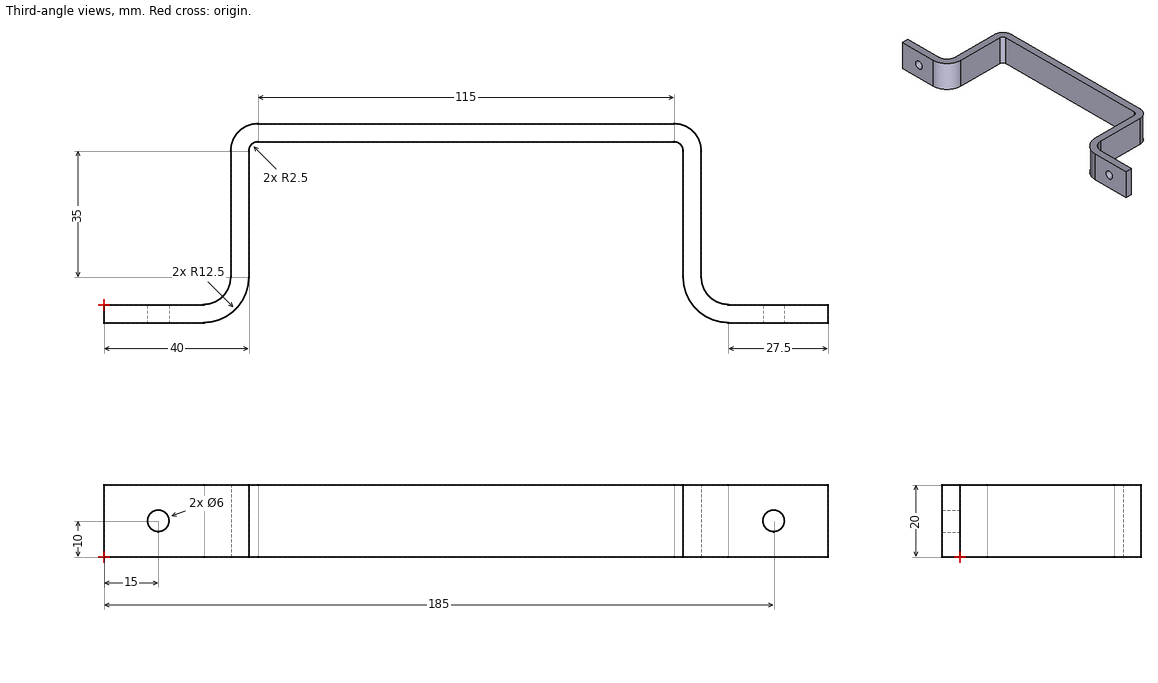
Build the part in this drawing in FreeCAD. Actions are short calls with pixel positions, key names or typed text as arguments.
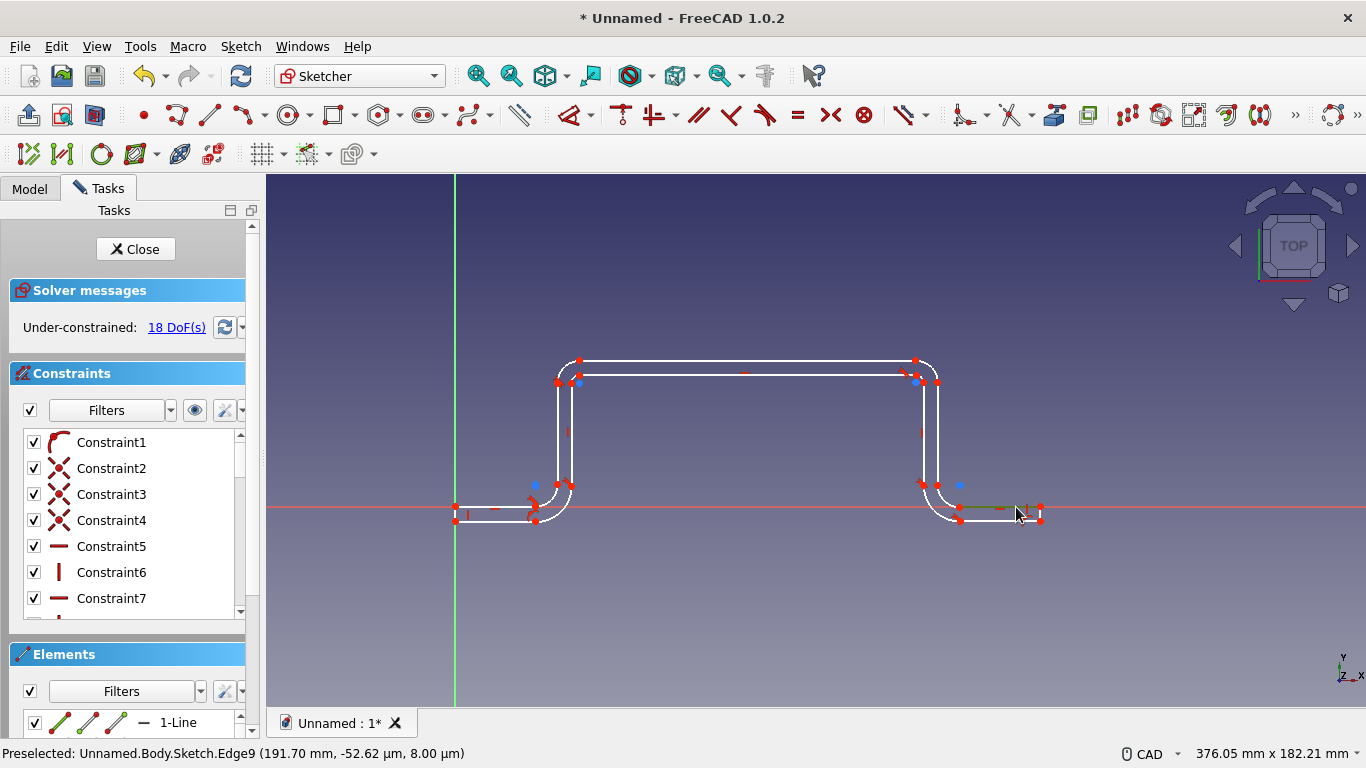
key(h)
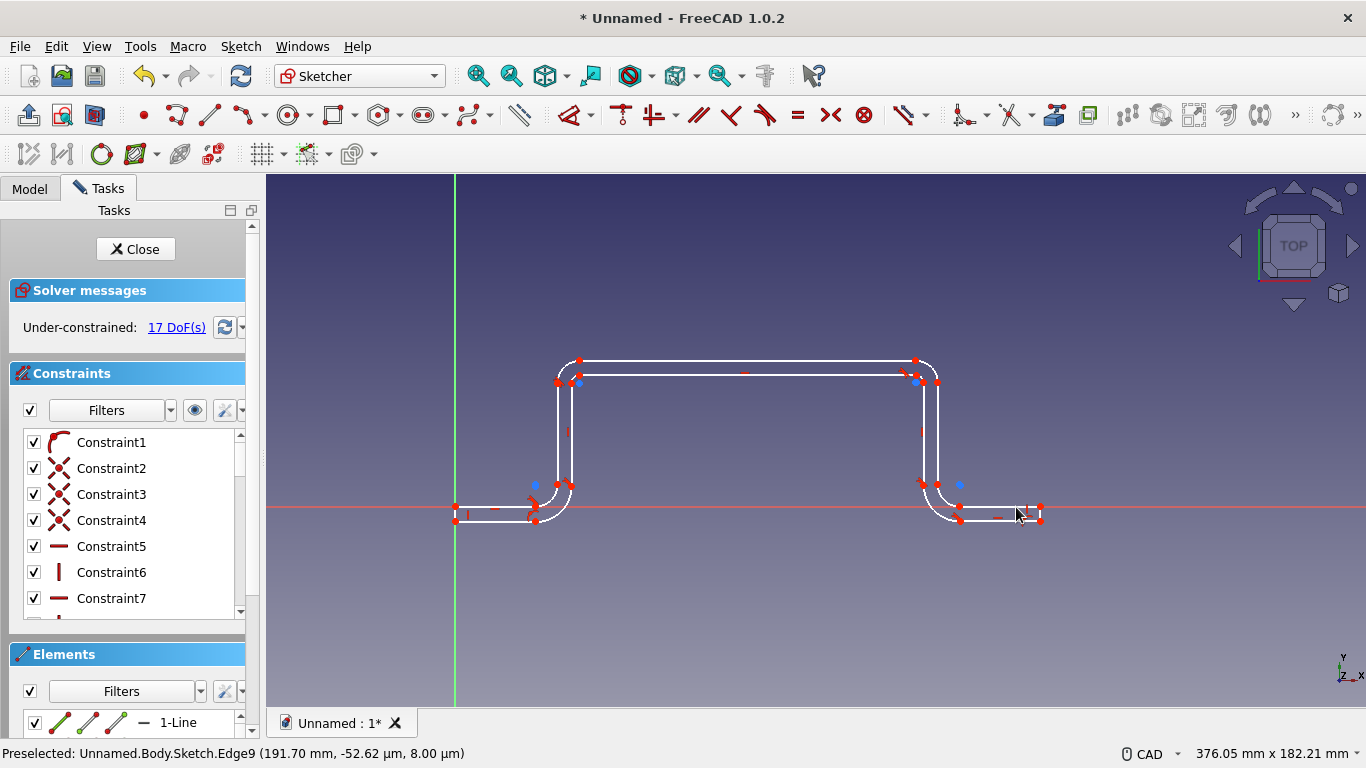
scroll(944, 518, up, 2)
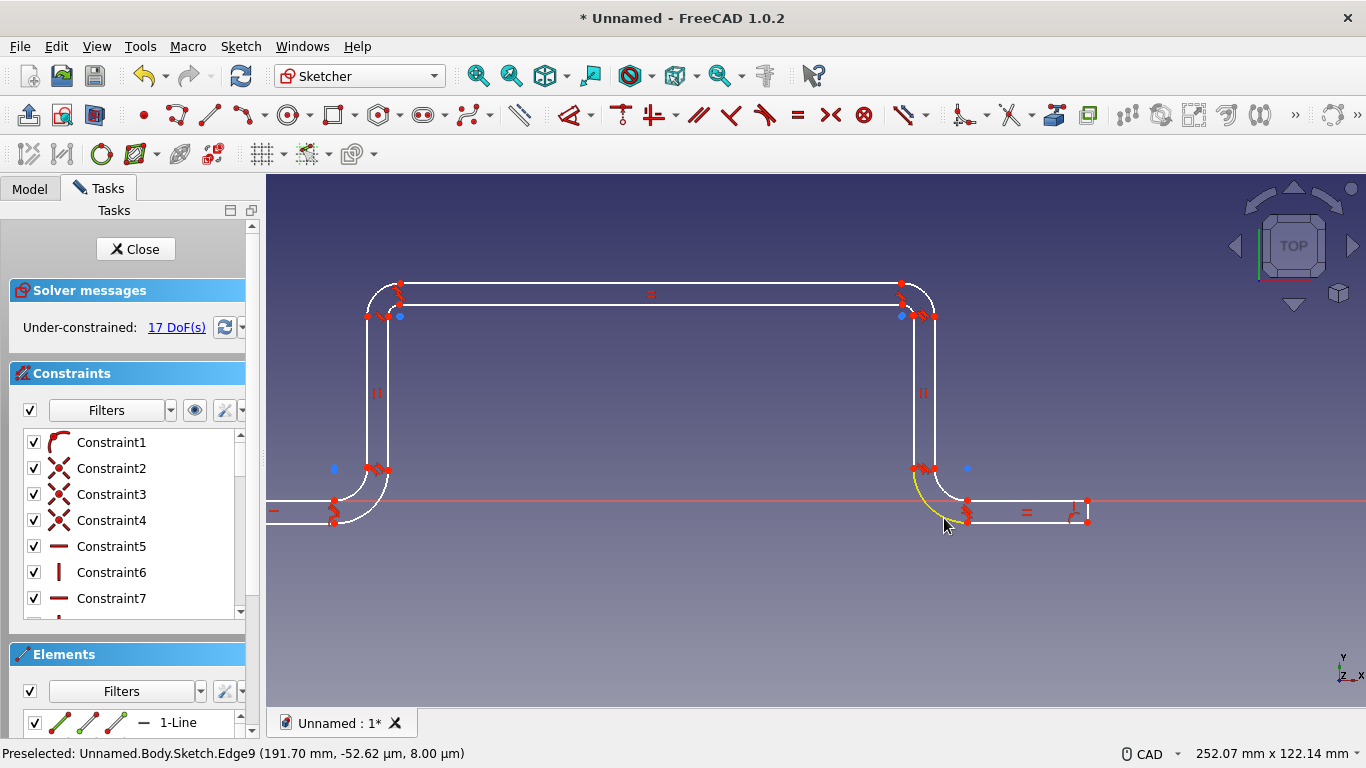
click(943, 517)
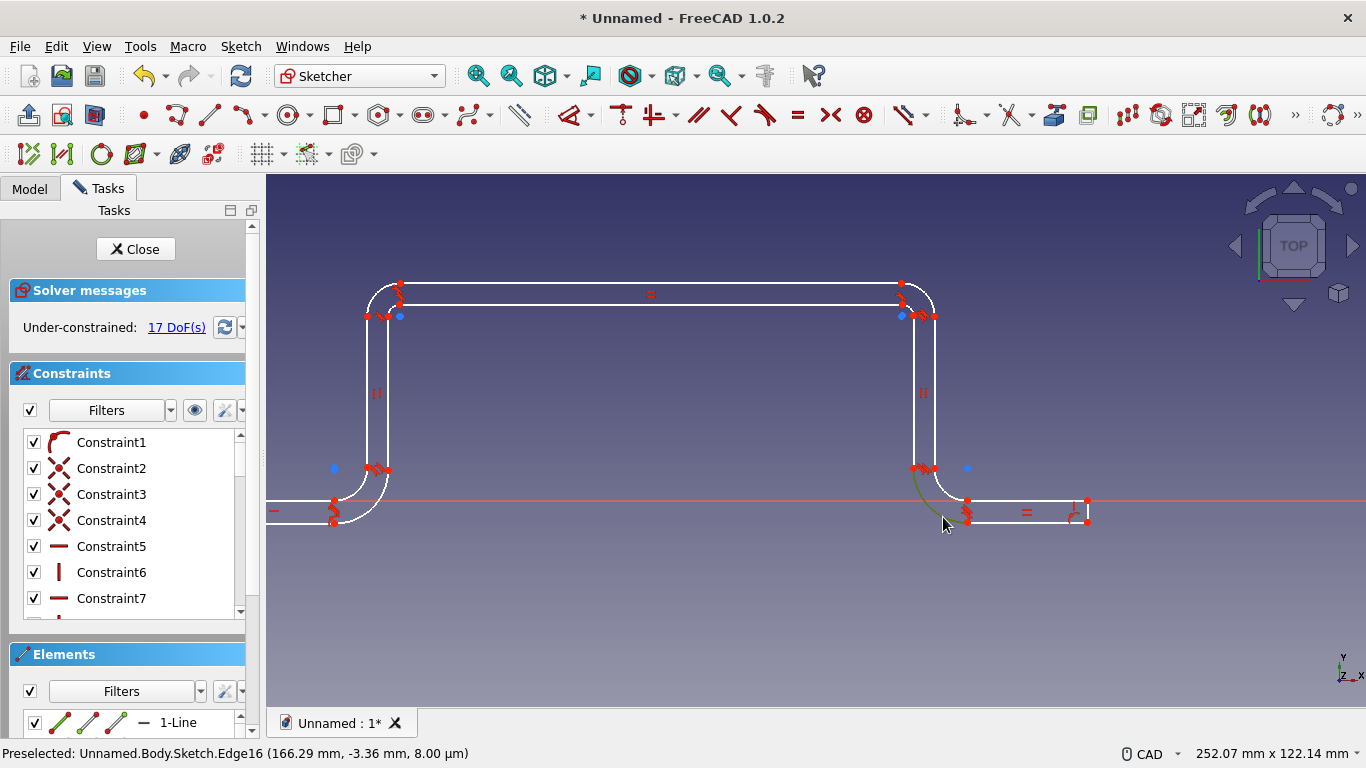
click(938, 483)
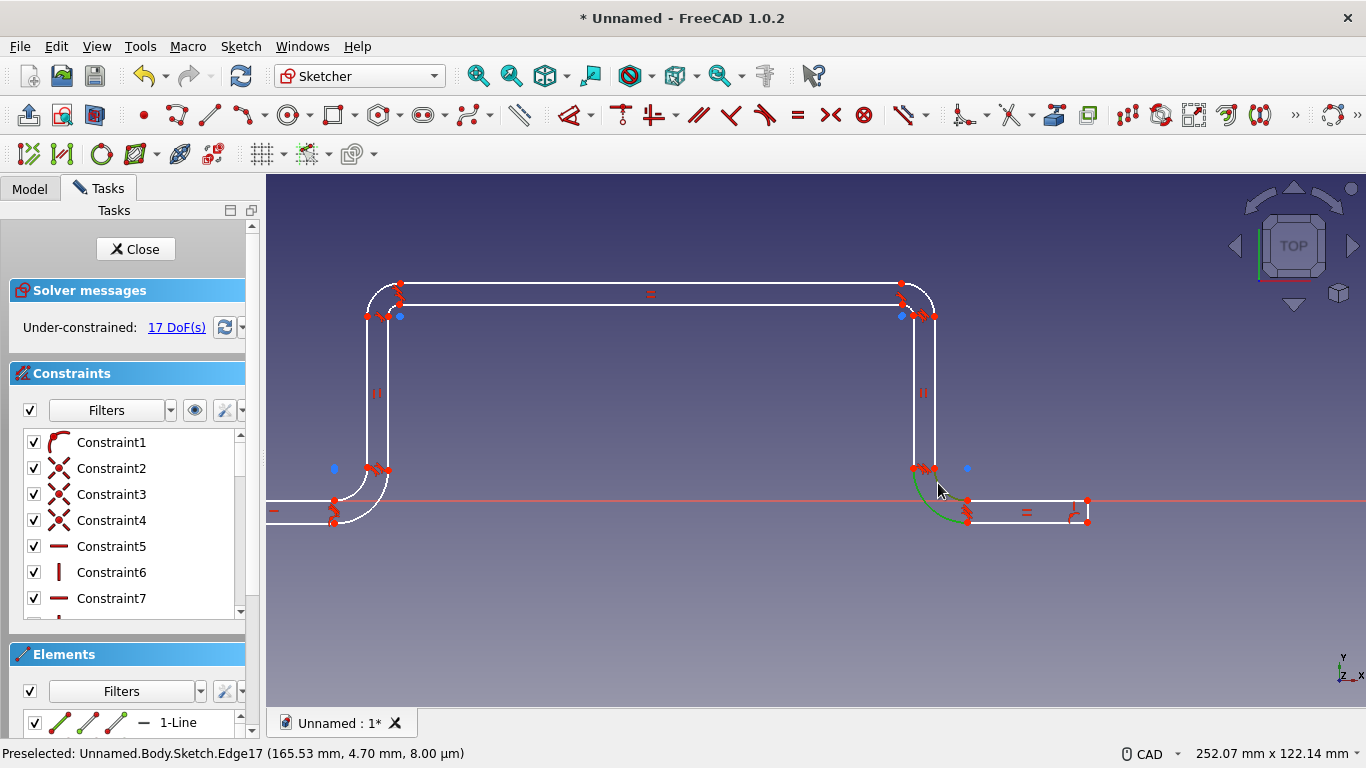
key(c)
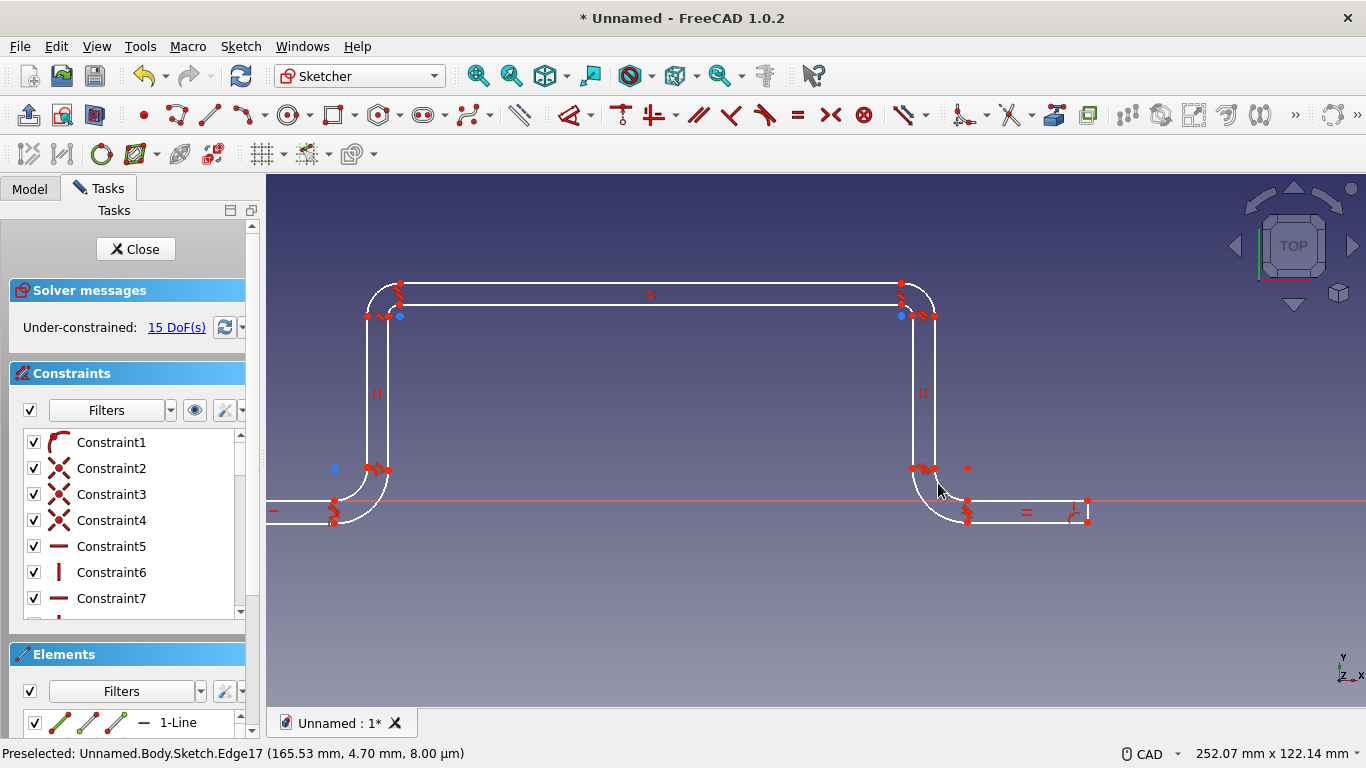
scroll(909, 308, up, 3)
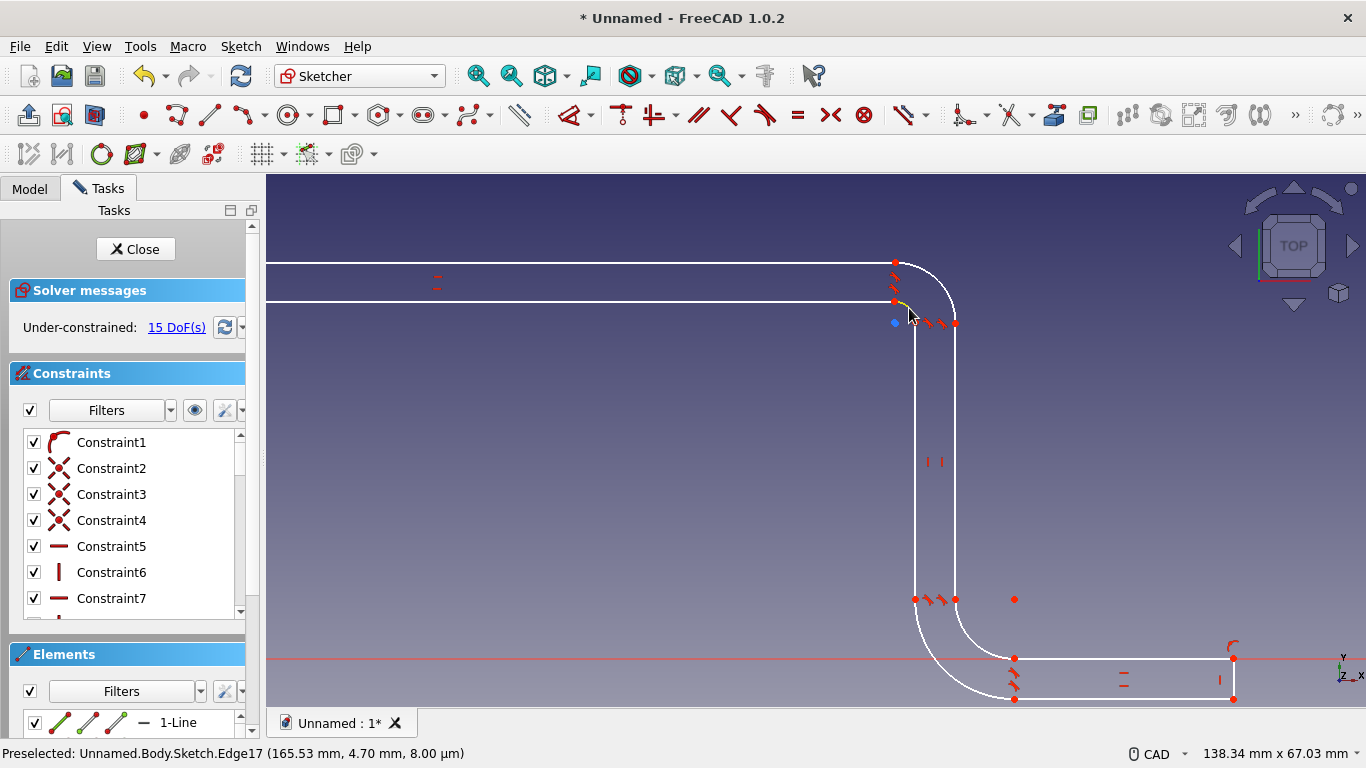
click(909, 308)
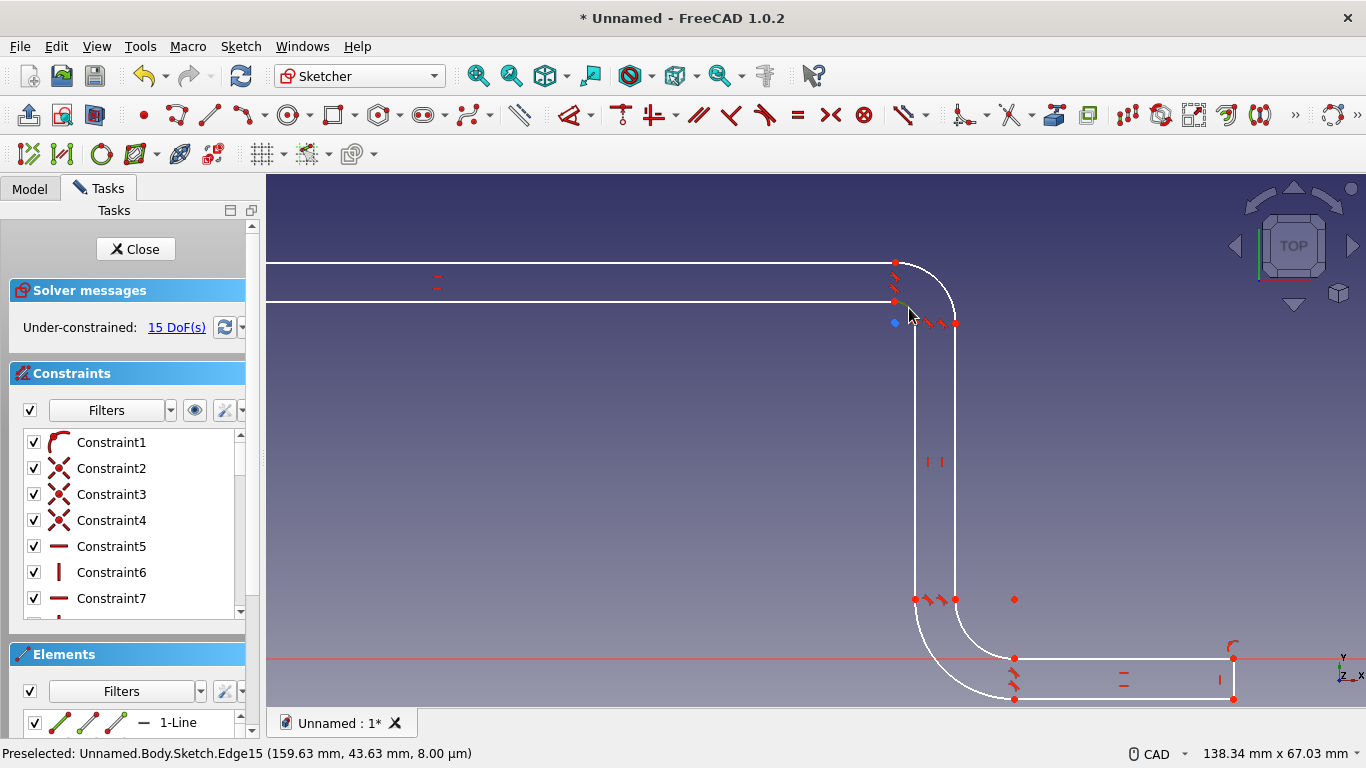
click(949, 296)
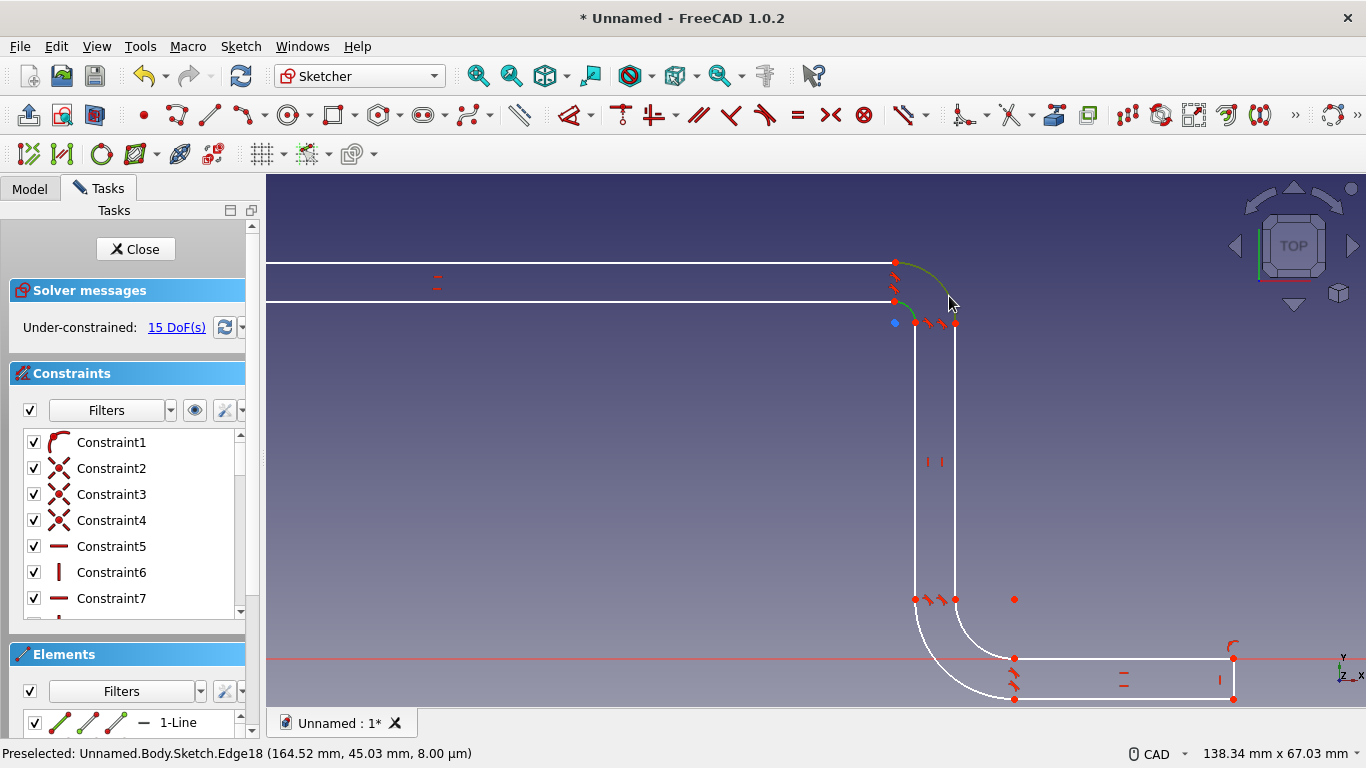
click(621, 116)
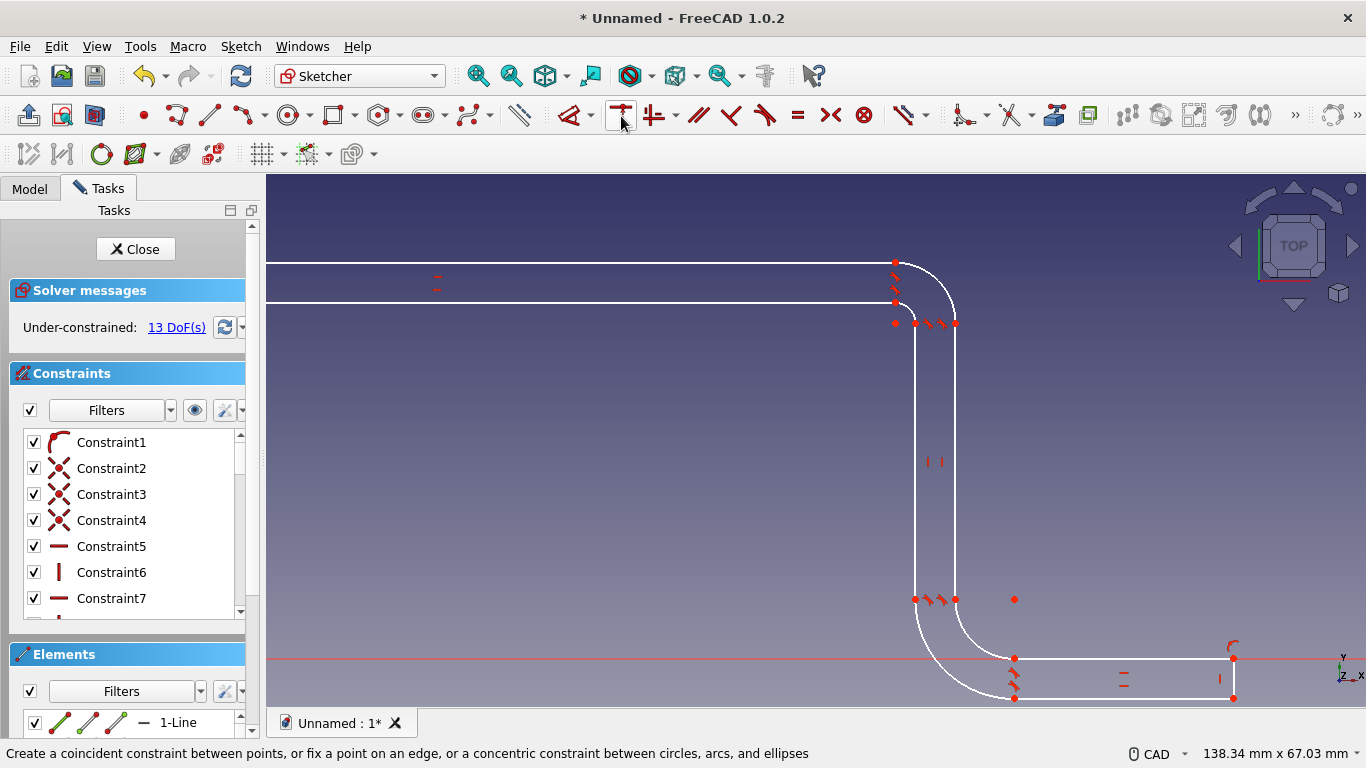
scroll(927, 418, down, 5)